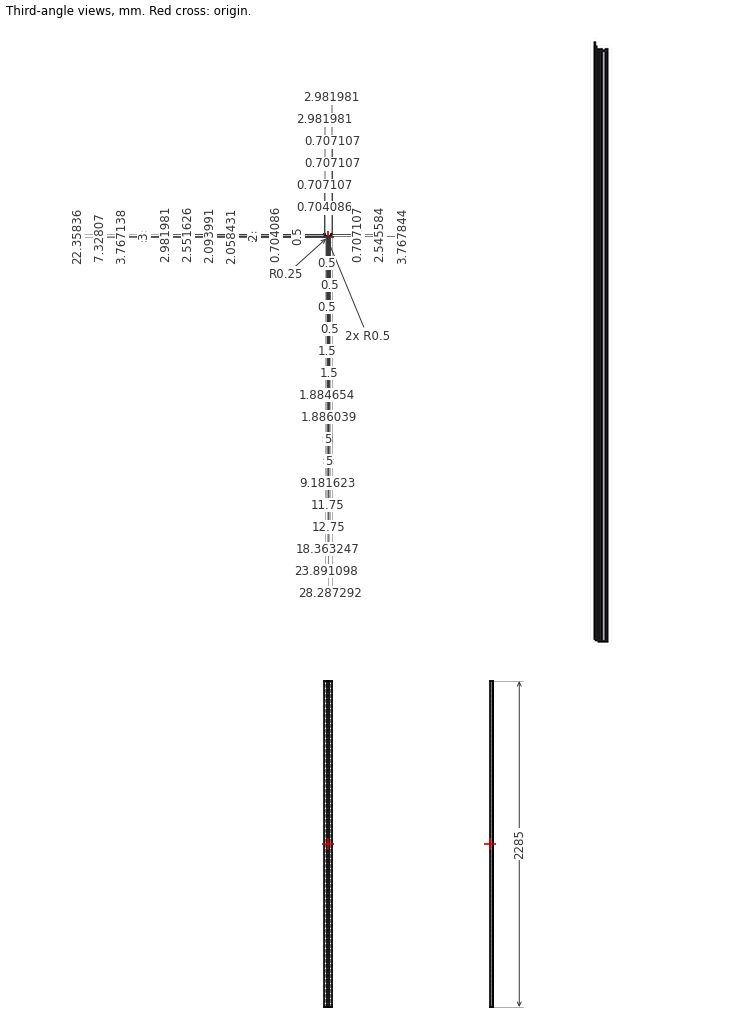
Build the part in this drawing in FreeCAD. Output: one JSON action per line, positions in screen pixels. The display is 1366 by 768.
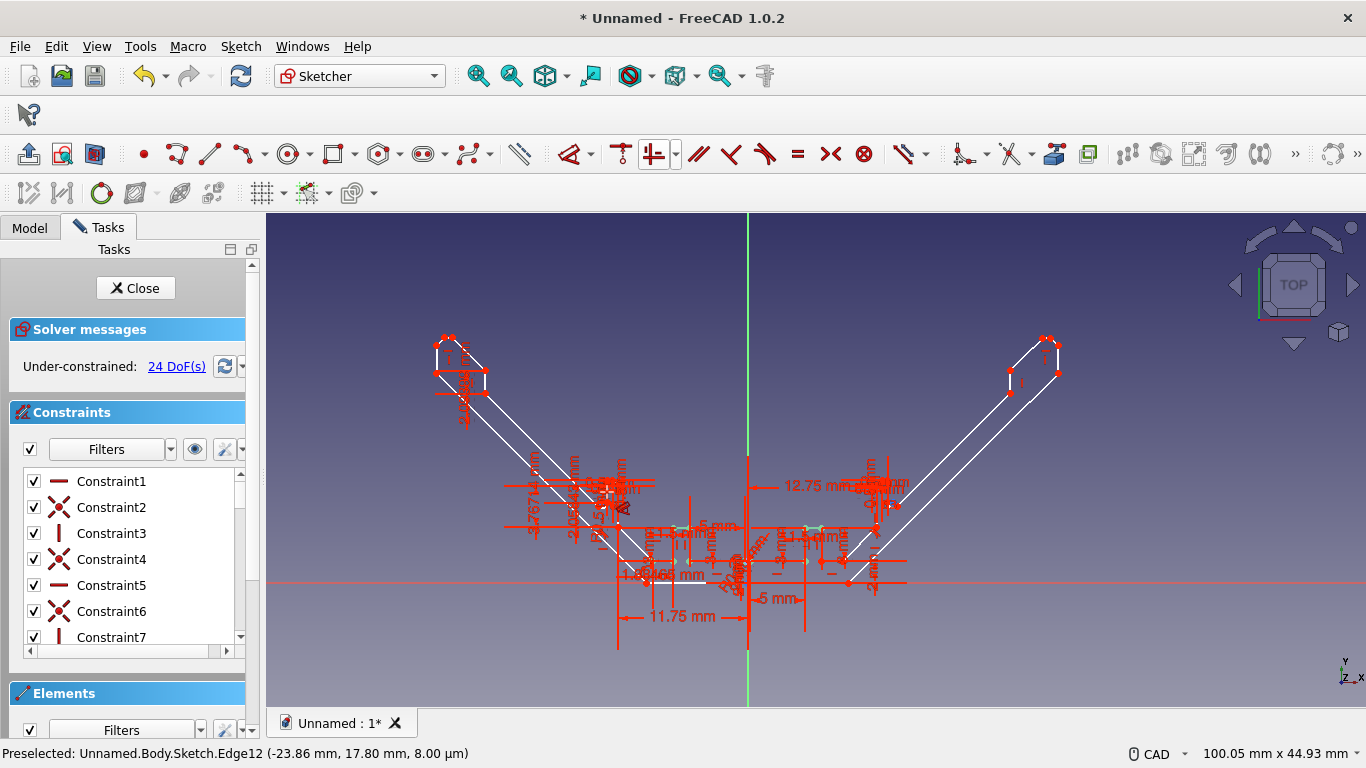
{"action": "scroll", "coordinate": [448, 338], "scroll_direction": "up", "scroll_amount": 9}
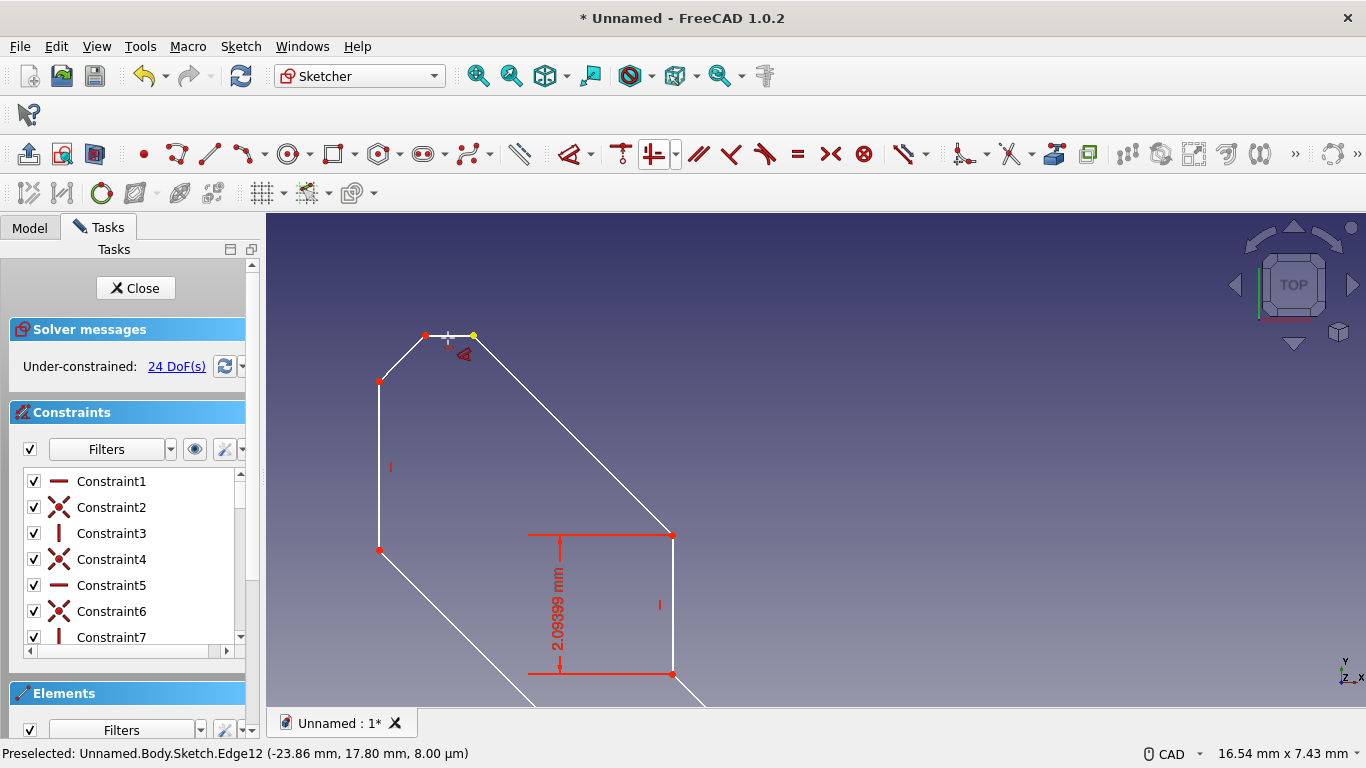
{"action": "left_click", "coordinate": [449, 336]}
{"action": "left_click", "coordinate": [449, 302]}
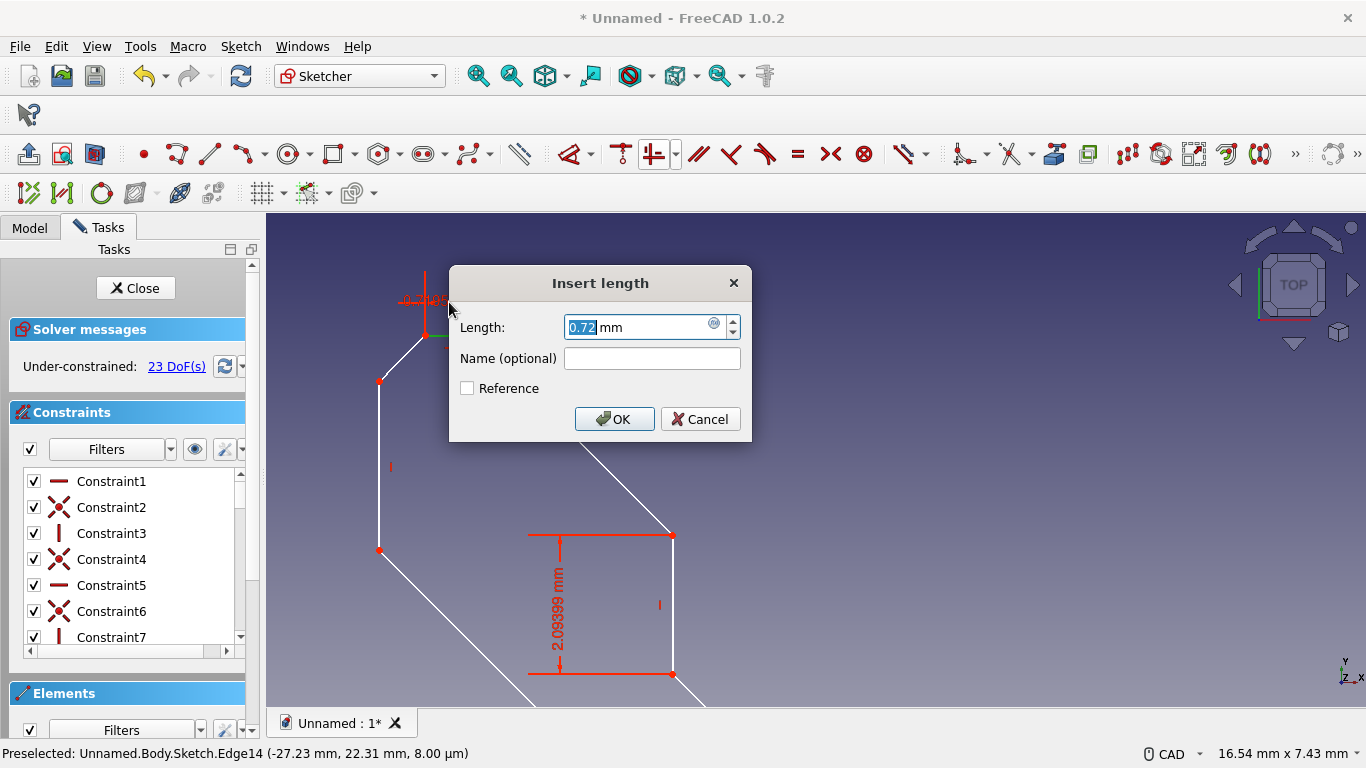
{"action": "type", "text": "0.707107"}
{"action": "key", "text": "Return"}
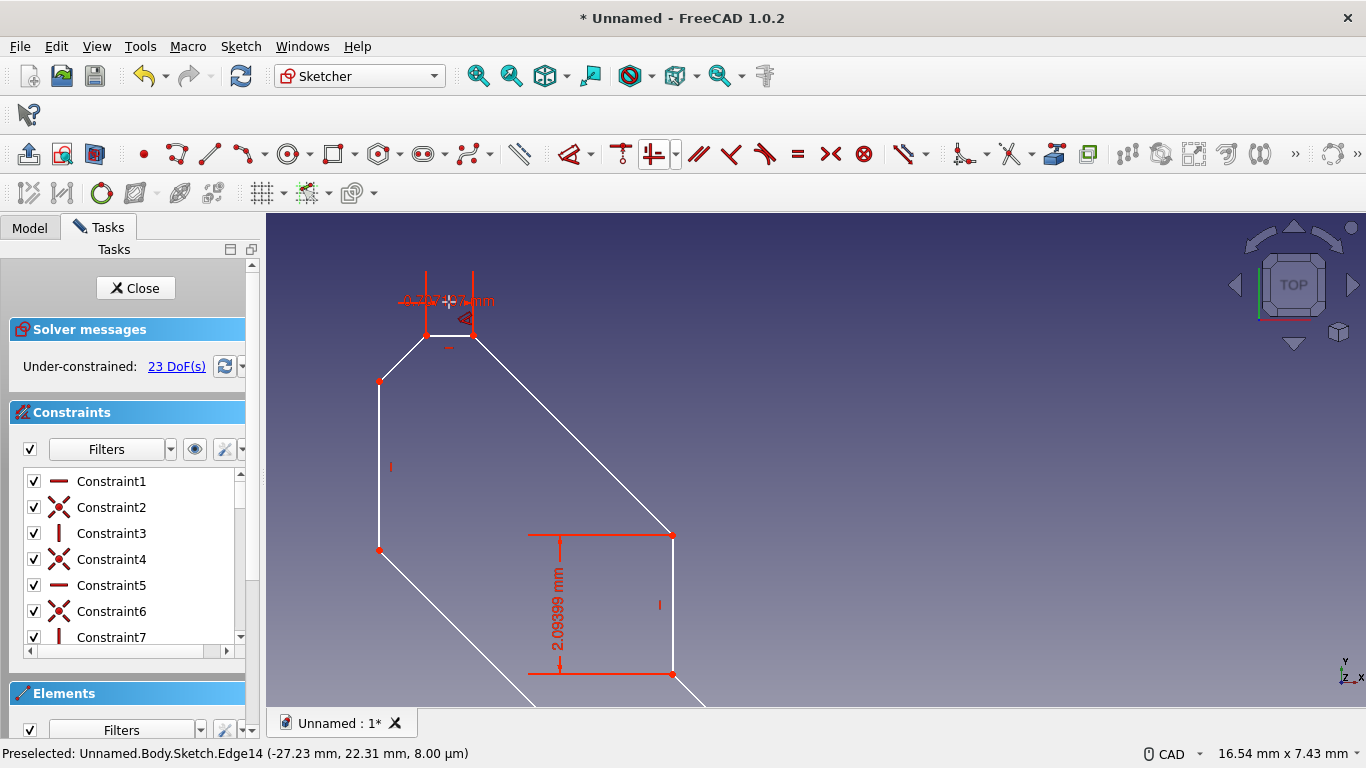
{"action": "scroll", "coordinate": [448, 338], "scroll_direction": "down", "scroll_amount": 9}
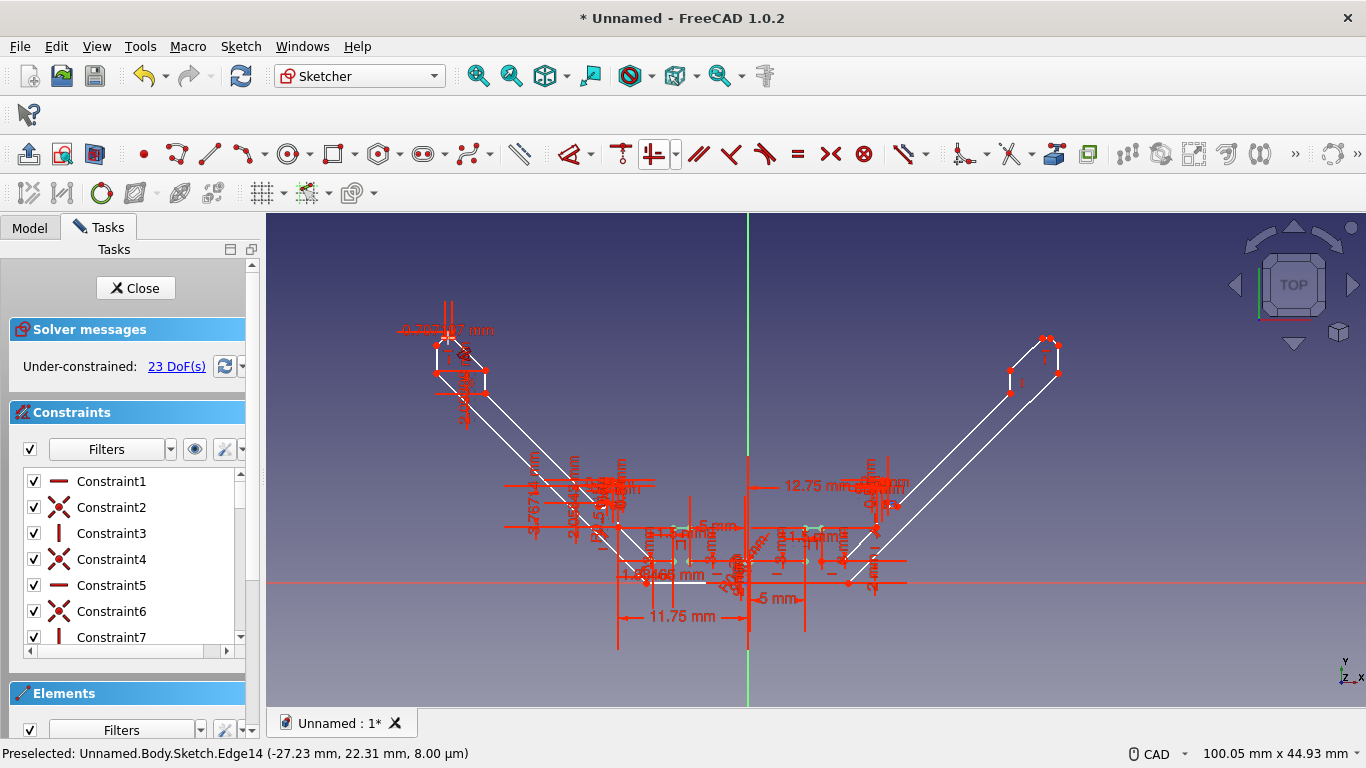
{"action": "scroll", "coordinate": [437, 354], "scroll_direction": "up", "scroll_amount": 3}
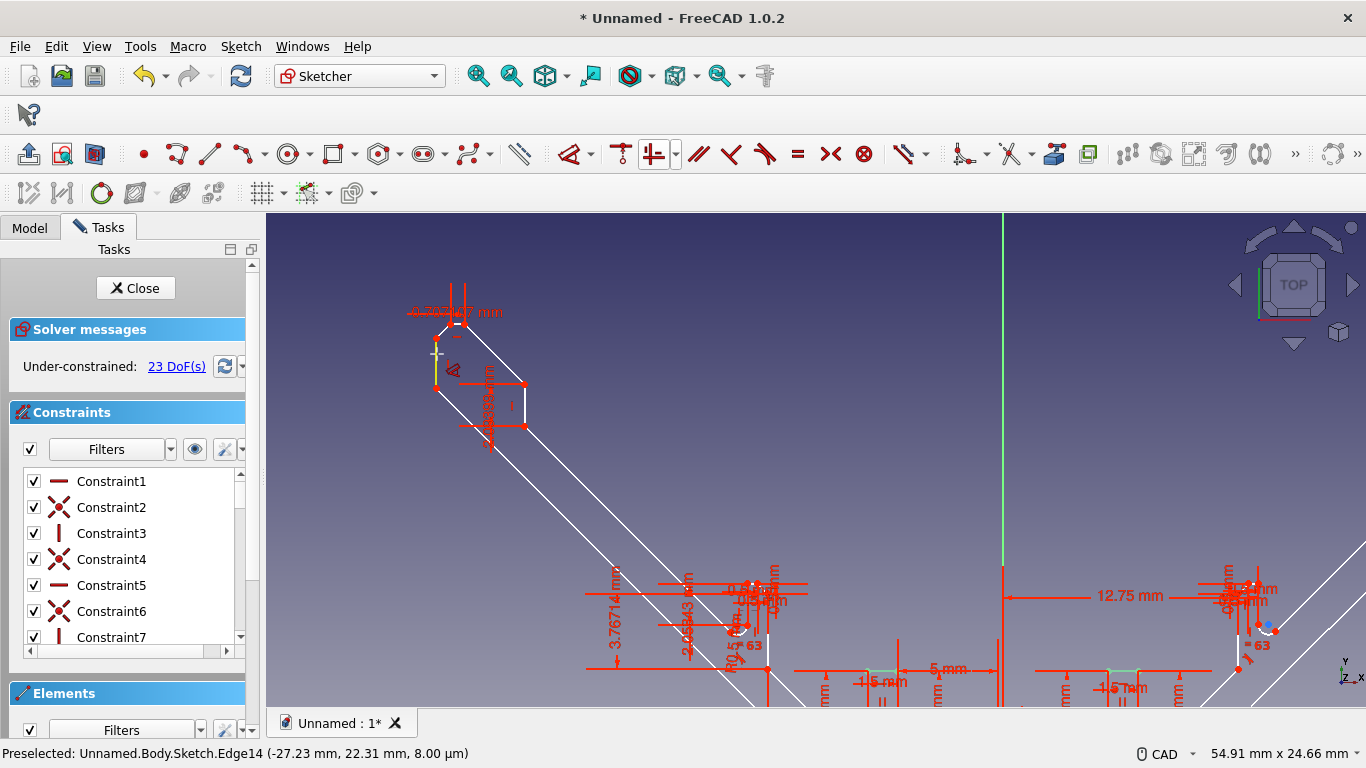
{"action": "left_click", "coordinate": [436, 353]}
{"action": "left_click", "coordinate": [402, 364]}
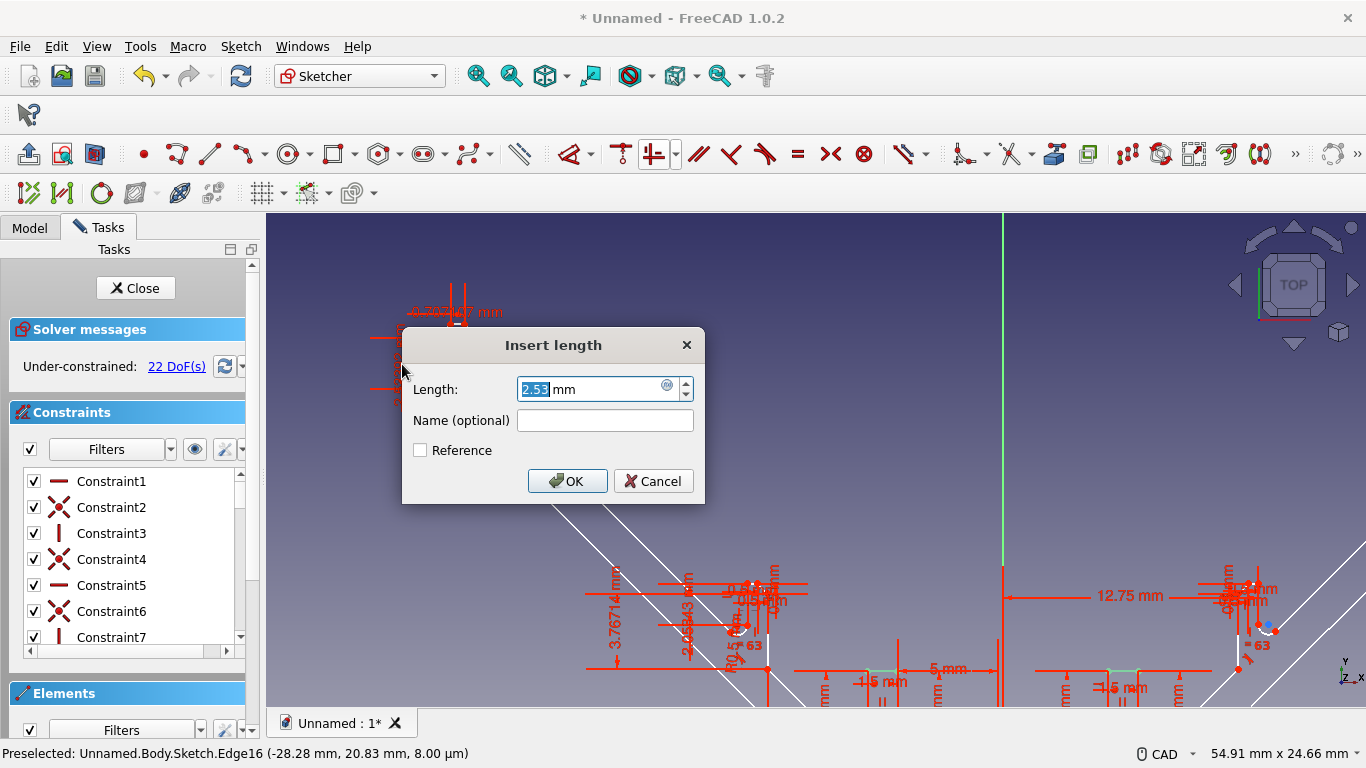
{"action": "type", "text": "2.551626"}
{"action": "key", "text": "Return"}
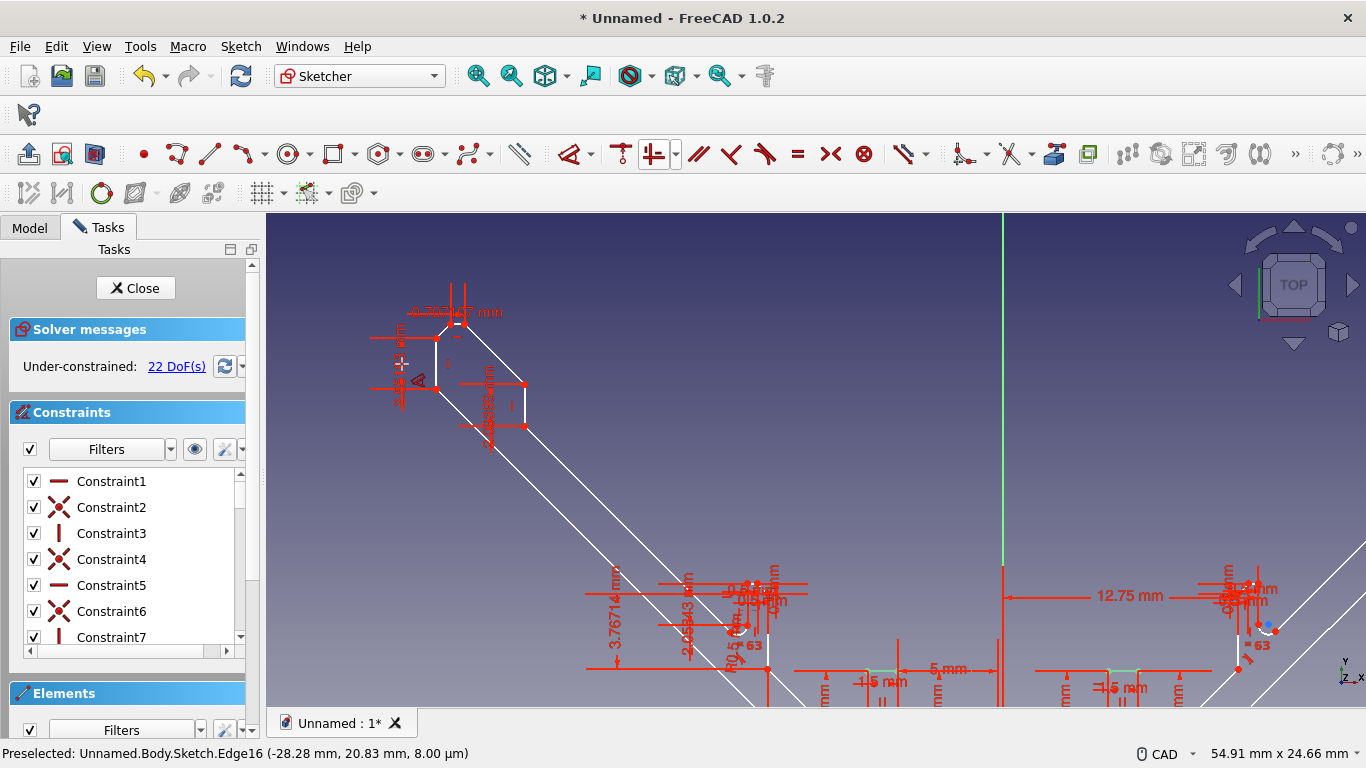
{"action": "scroll", "coordinate": [437, 354], "scroll_direction": "down", "scroll_amount": 3}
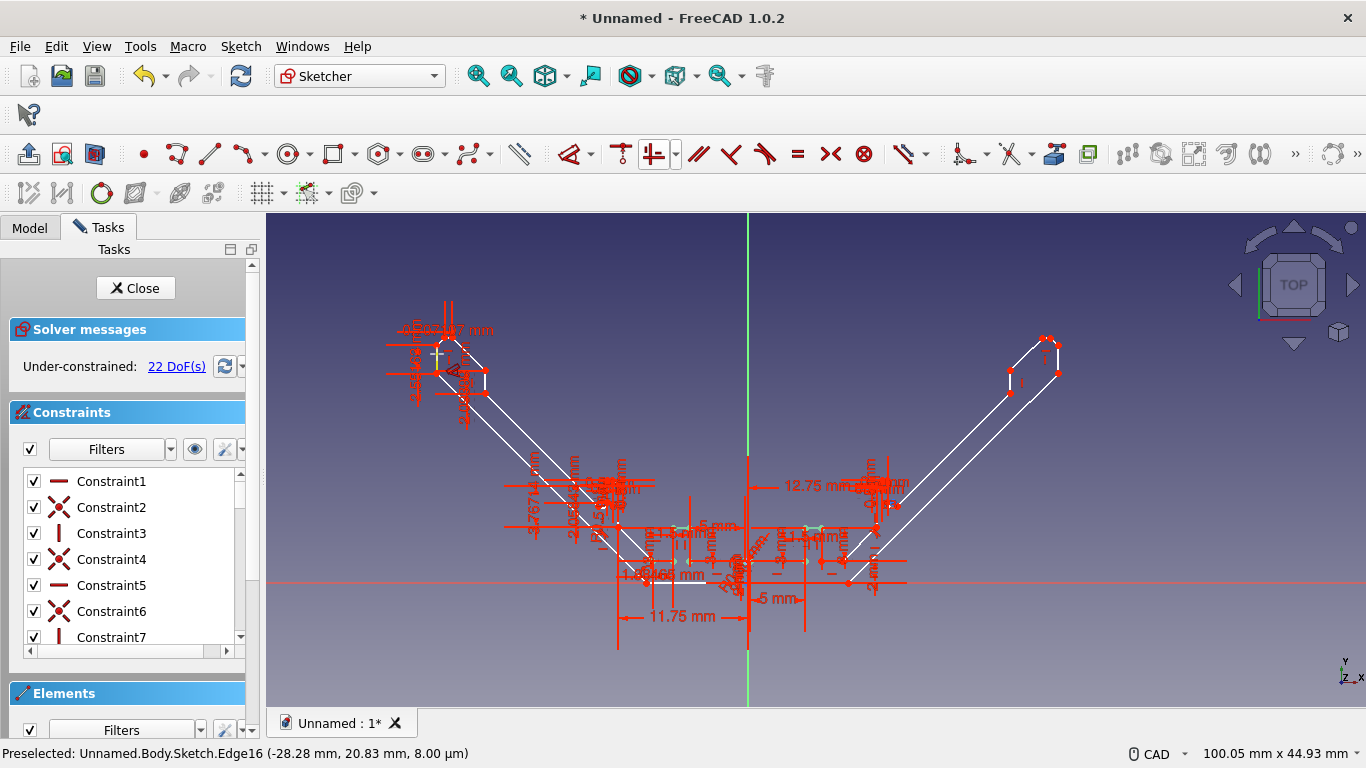
{"action": "scroll", "coordinate": [1058, 365], "scroll_direction": "up", "scroll_amount": 3}